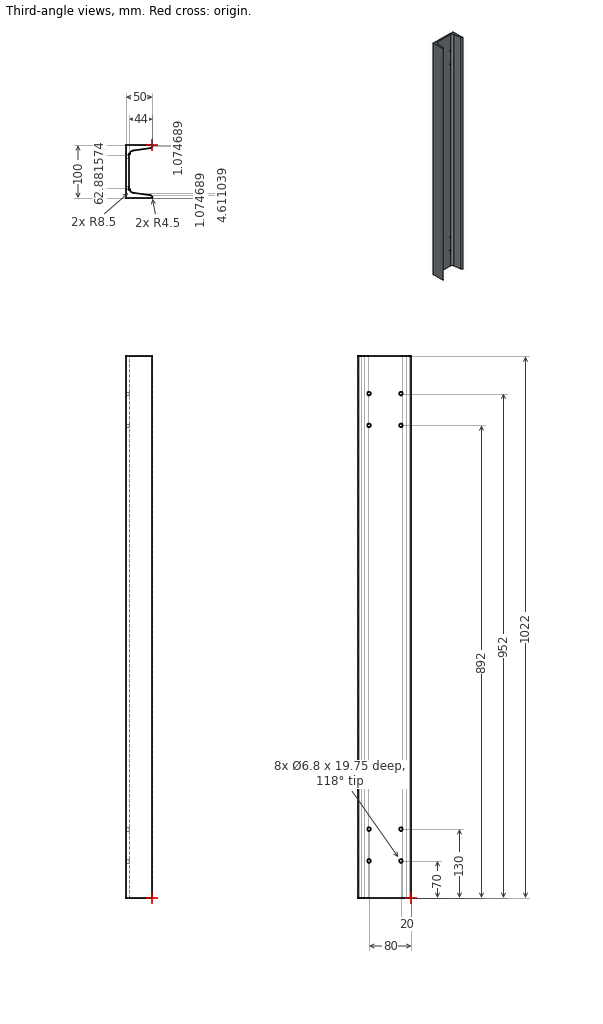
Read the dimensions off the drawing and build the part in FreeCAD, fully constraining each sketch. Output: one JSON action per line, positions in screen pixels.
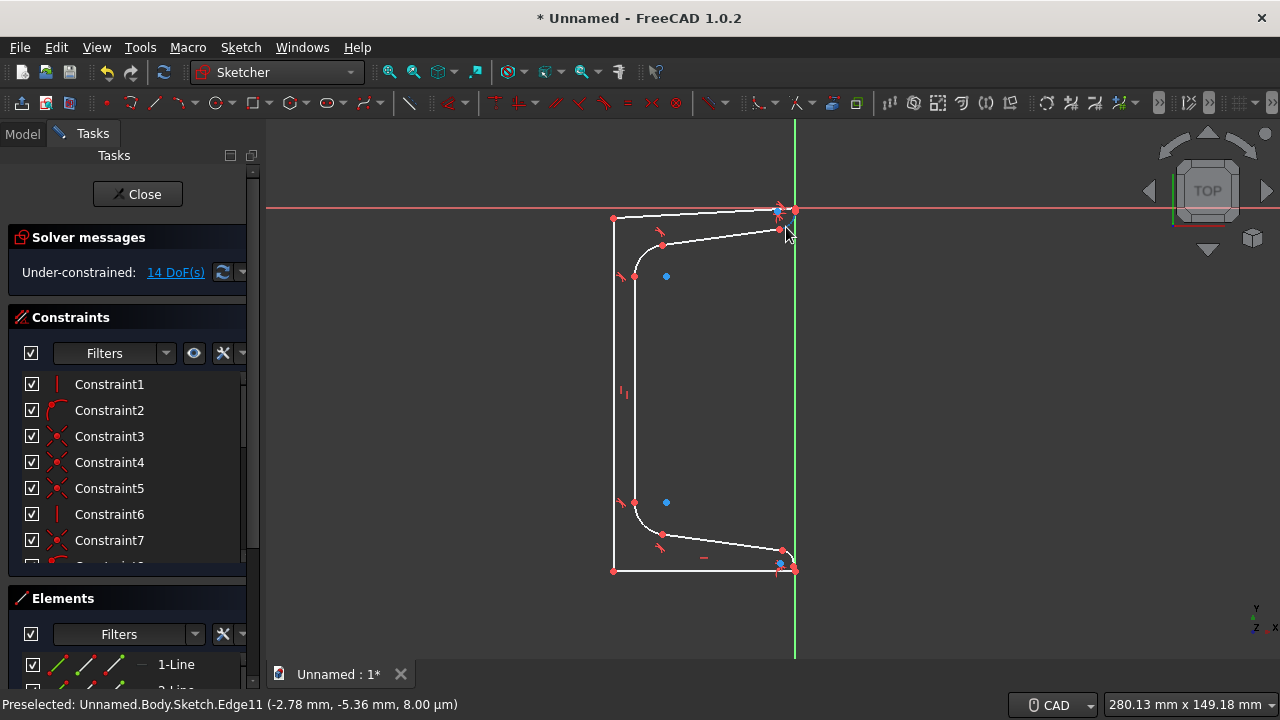
{"action": "scroll", "coordinate": [794, 569], "scroll_direction": "up", "scroll_amount": 10}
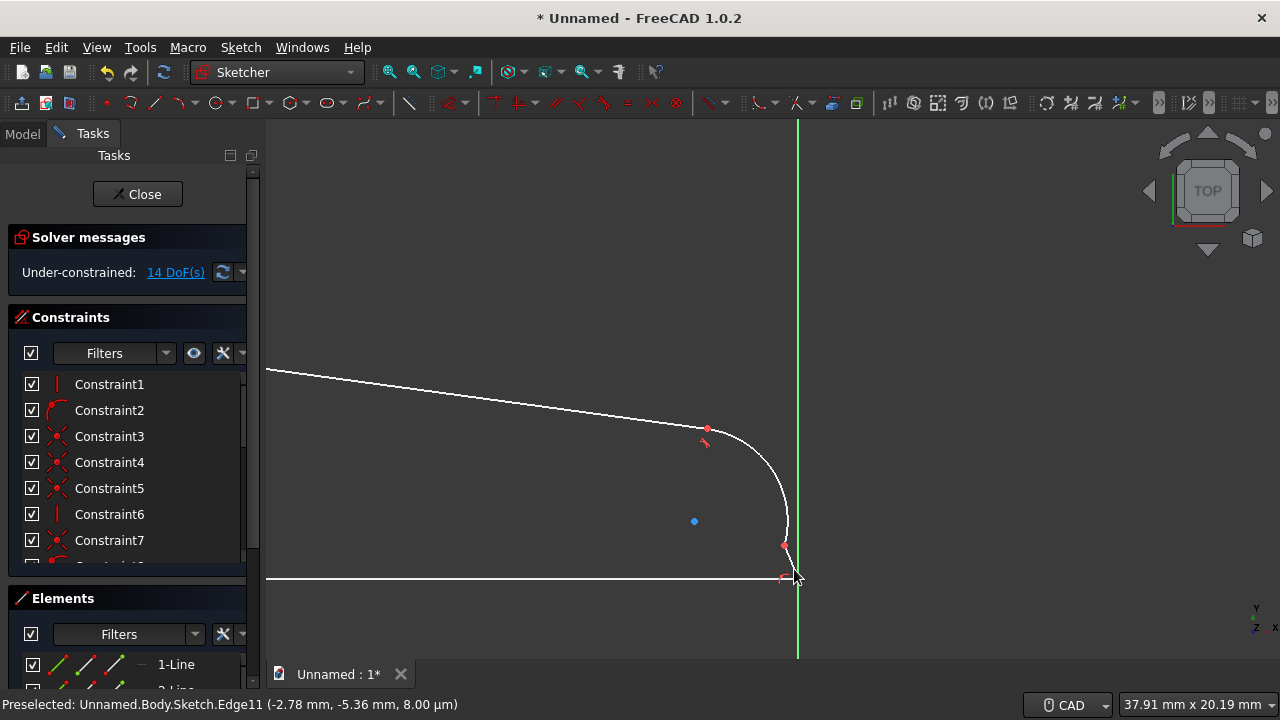
{"action": "left_click", "coordinate": [791, 562]}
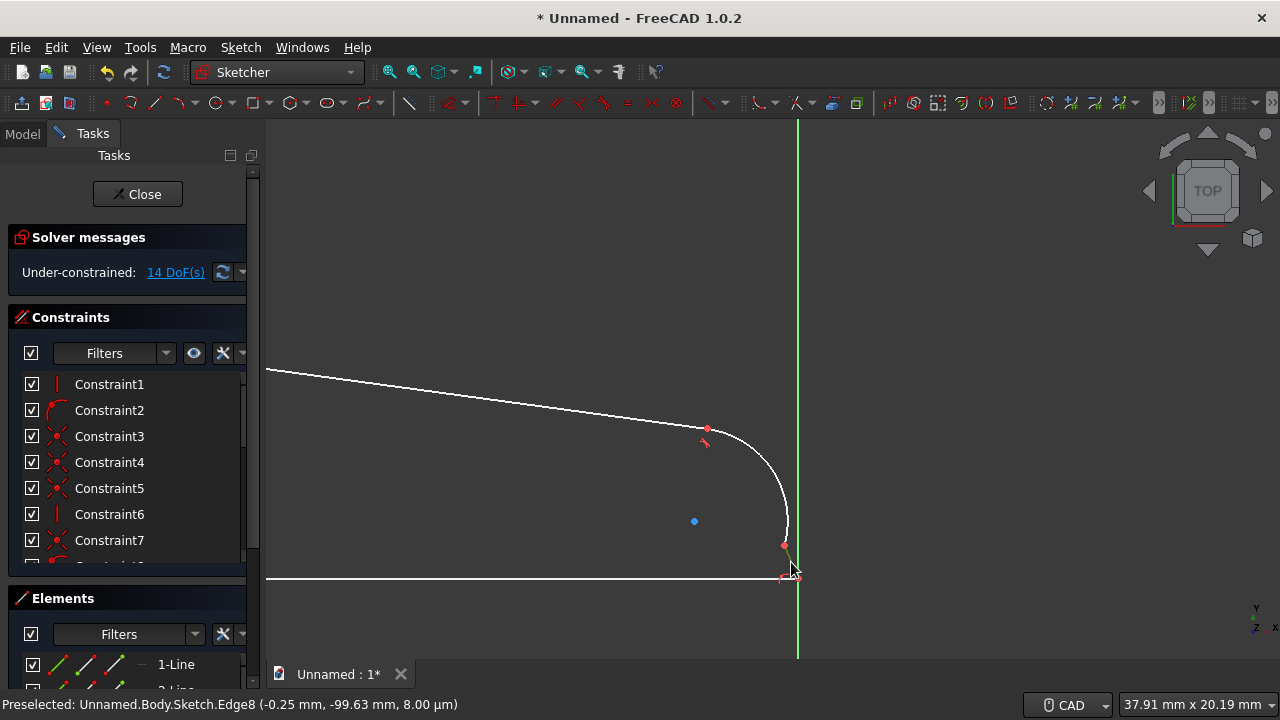
{"action": "left_click", "coordinate": [785, 499]}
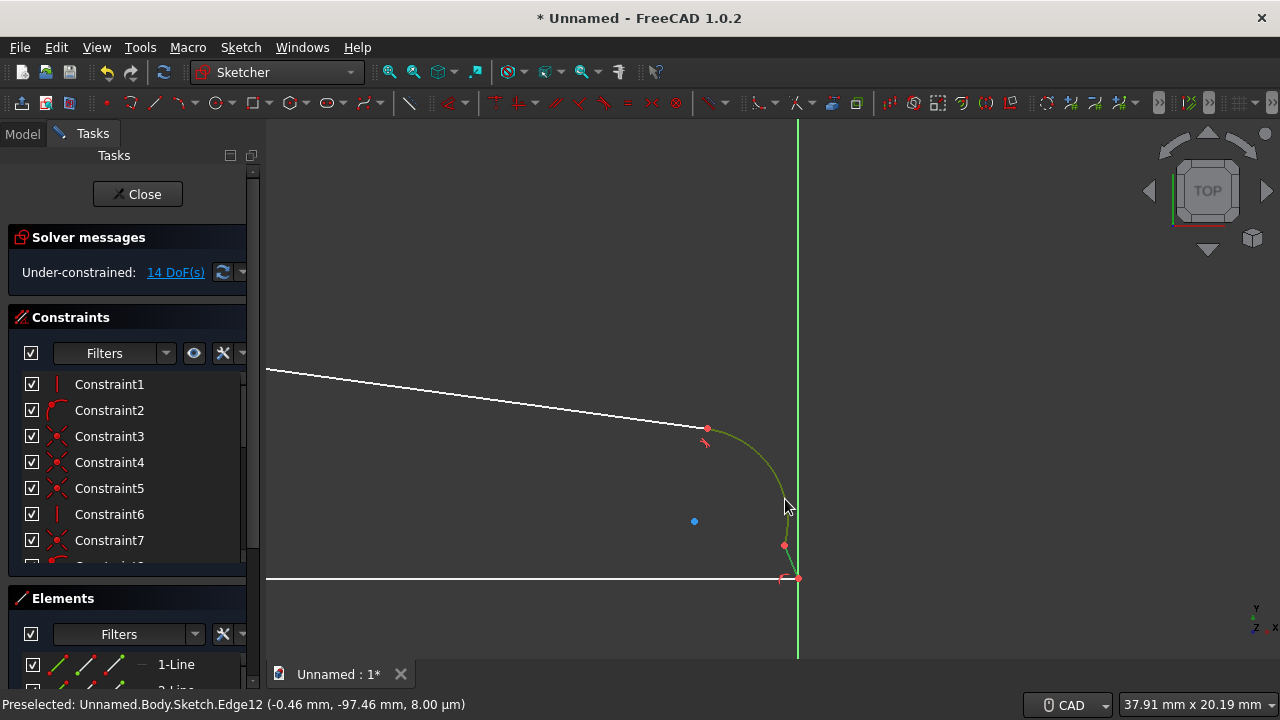
{"action": "left_click", "coordinate": [604, 104]}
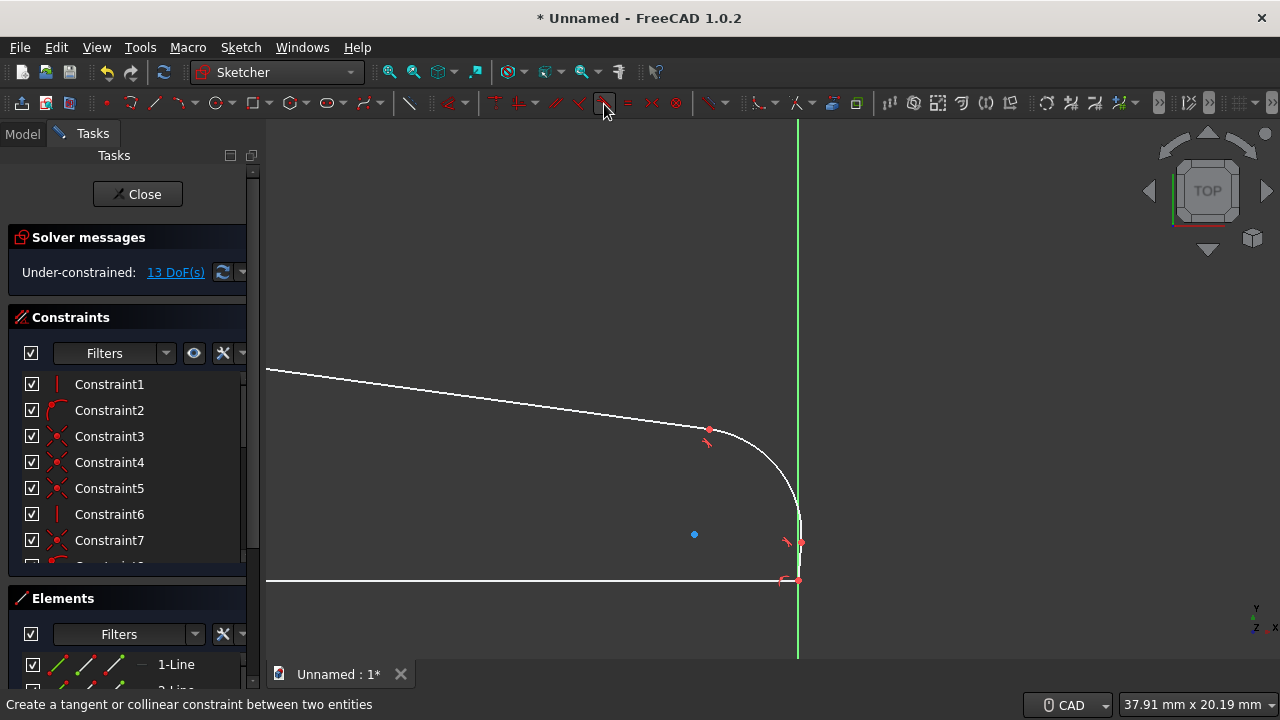
{"action": "scroll", "coordinate": [794, 570], "scroll_direction": "down", "scroll_amount": 10}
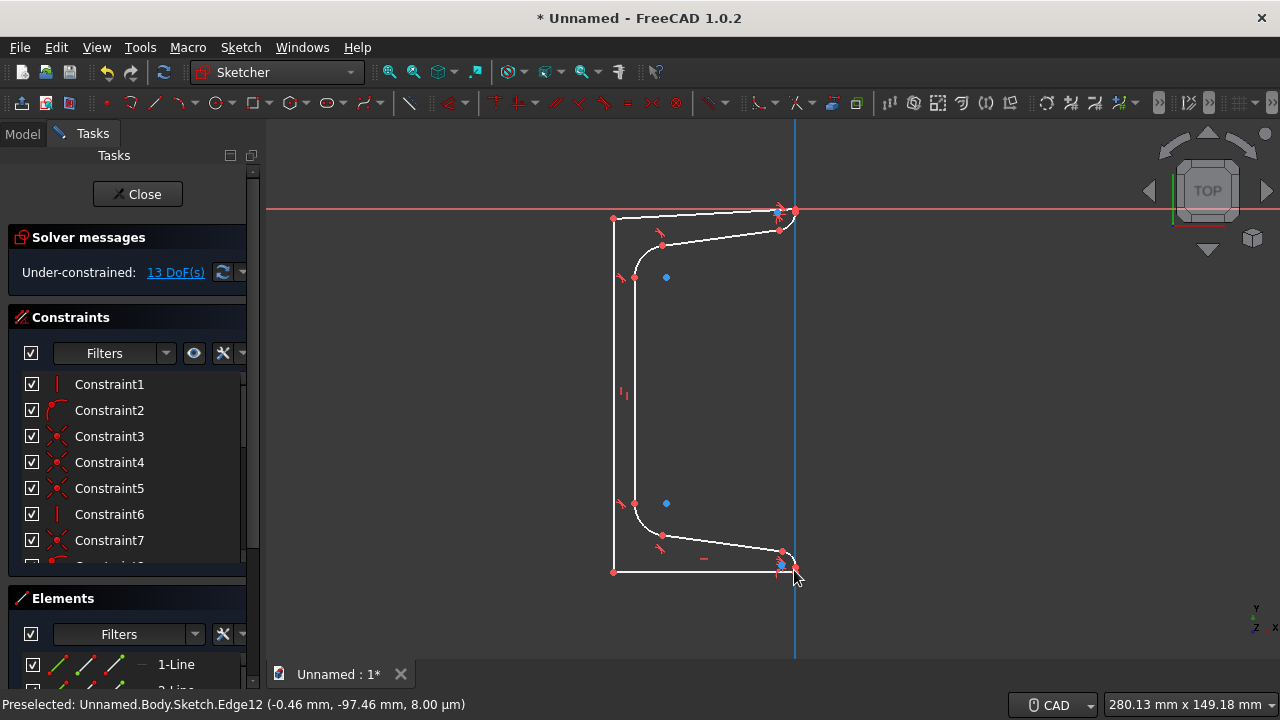
{"action": "scroll", "coordinate": [741, 212], "scroll_direction": "up", "scroll_amount": 8}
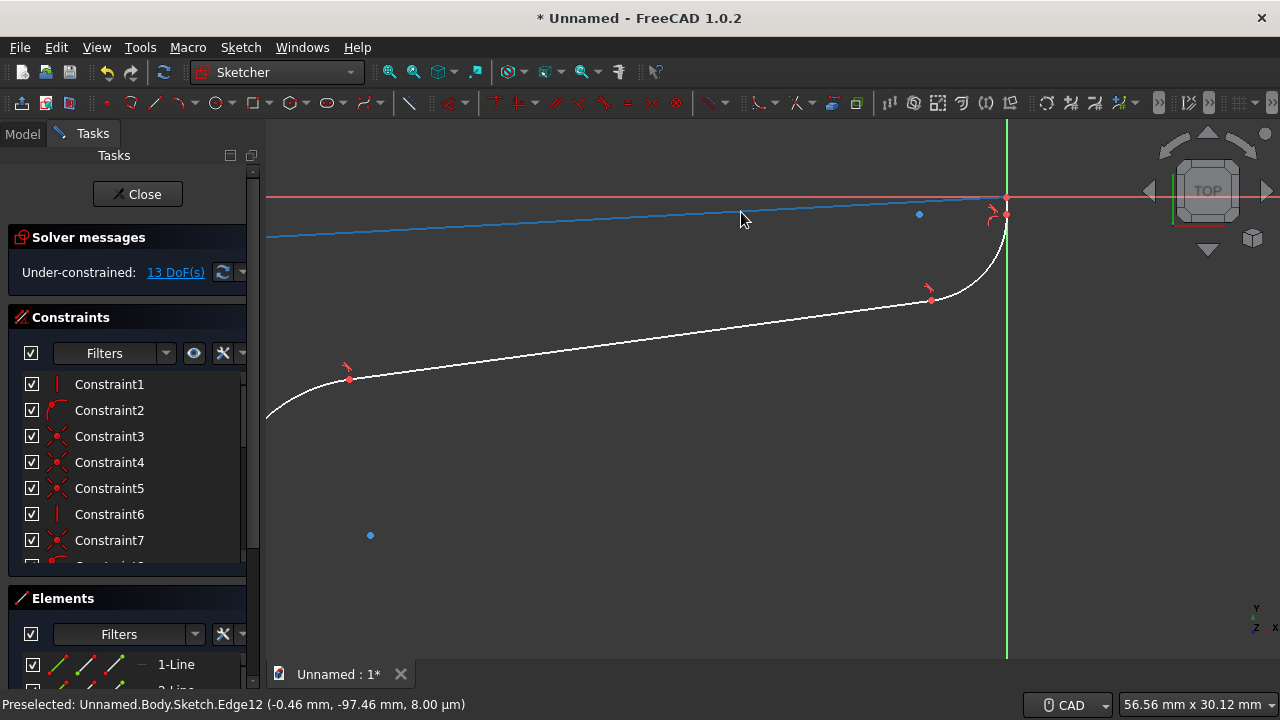
{"action": "left_click", "coordinate": [738, 212]}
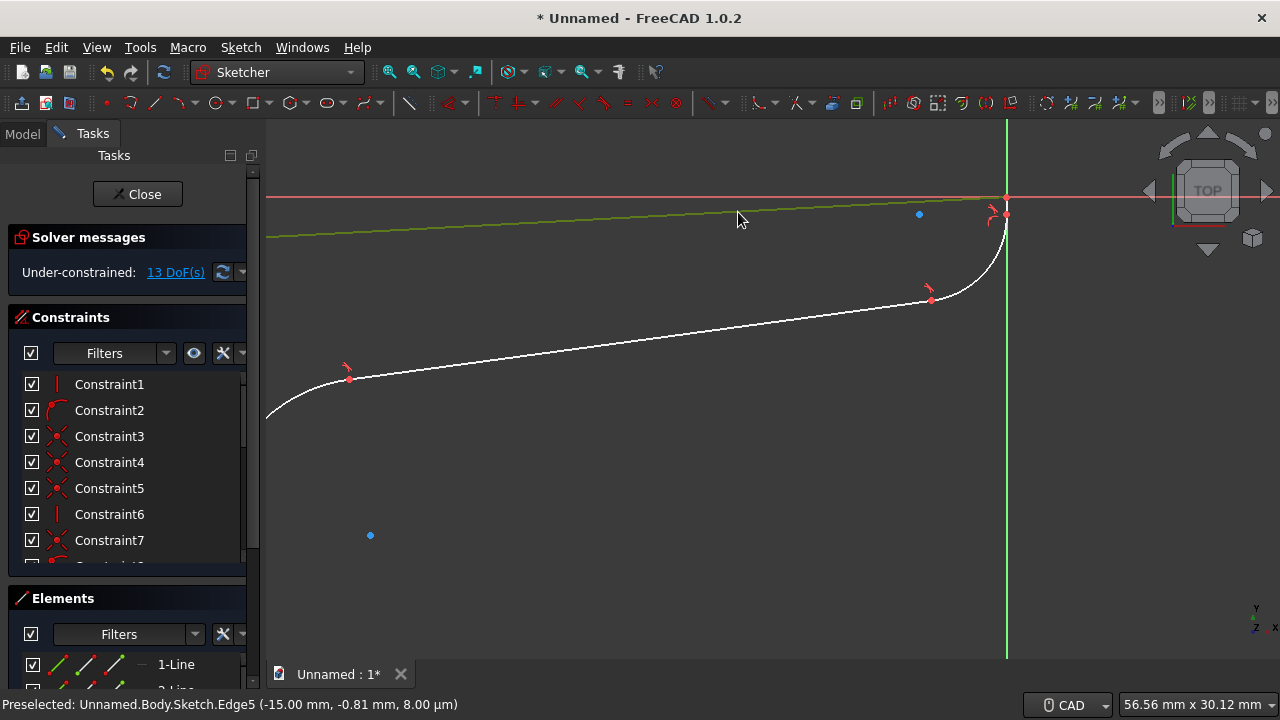
{"action": "key", "text": "h"}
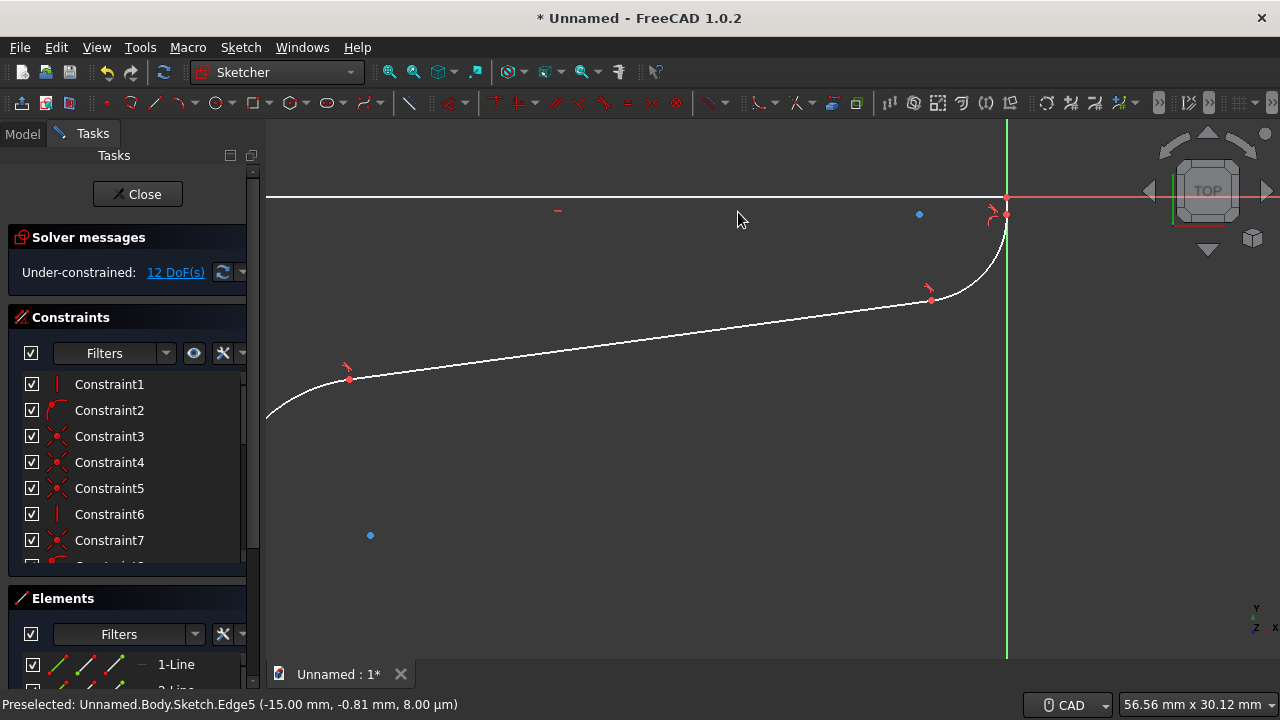
{"action": "scroll", "coordinate": [741, 211], "scroll_direction": "down", "scroll_amount": 8}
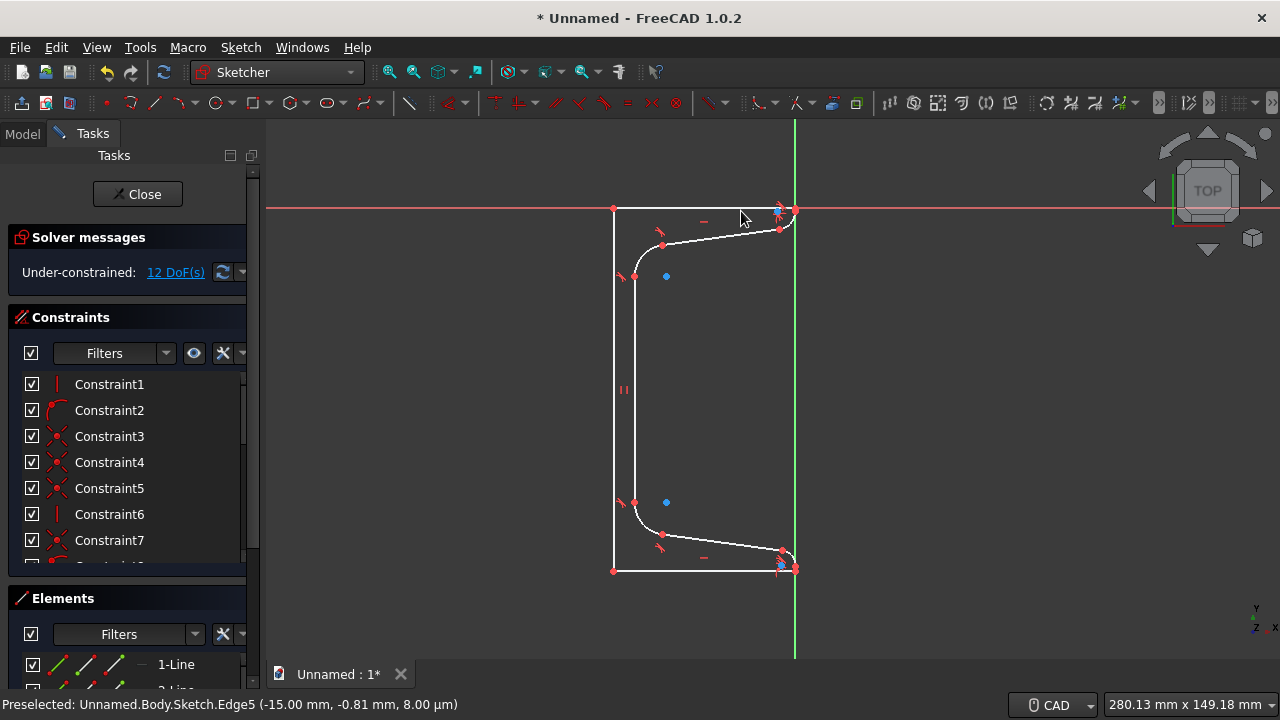
{"action": "scroll", "coordinate": [795, 569], "scroll_direction": "up", "scroll_amount": 10}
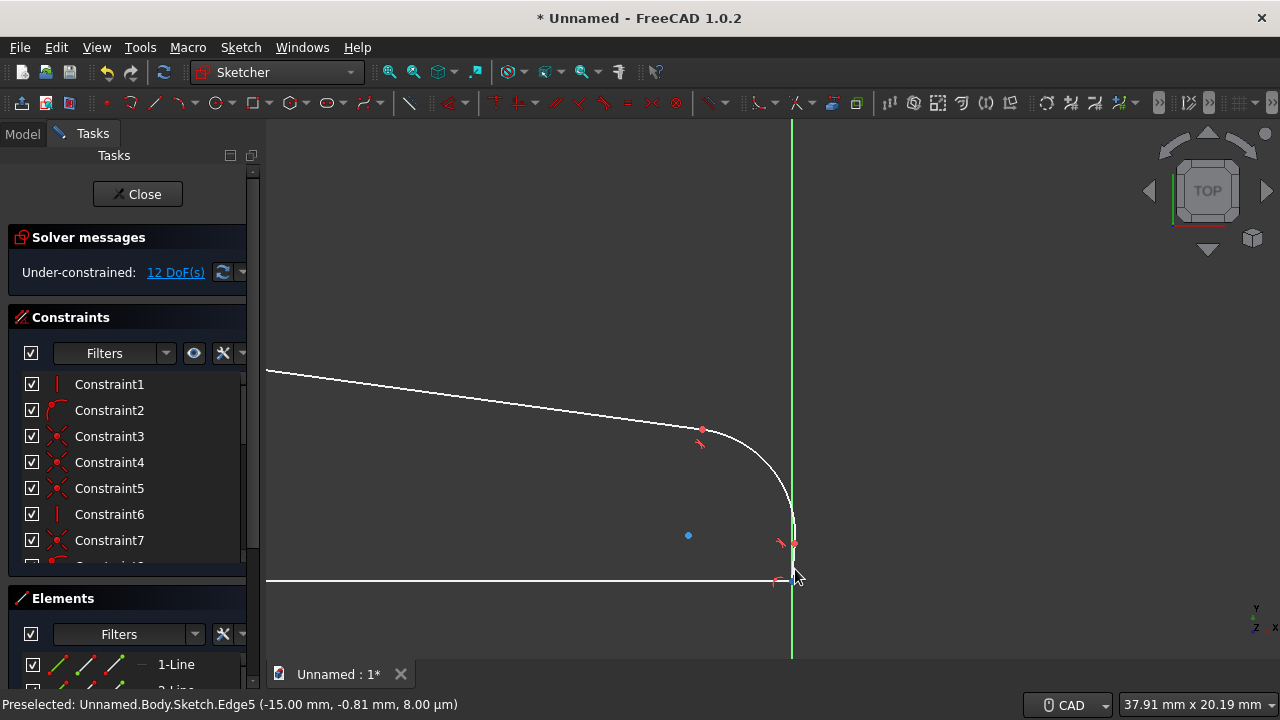
{"action": "left_click", "coordinate": [793, 566]}